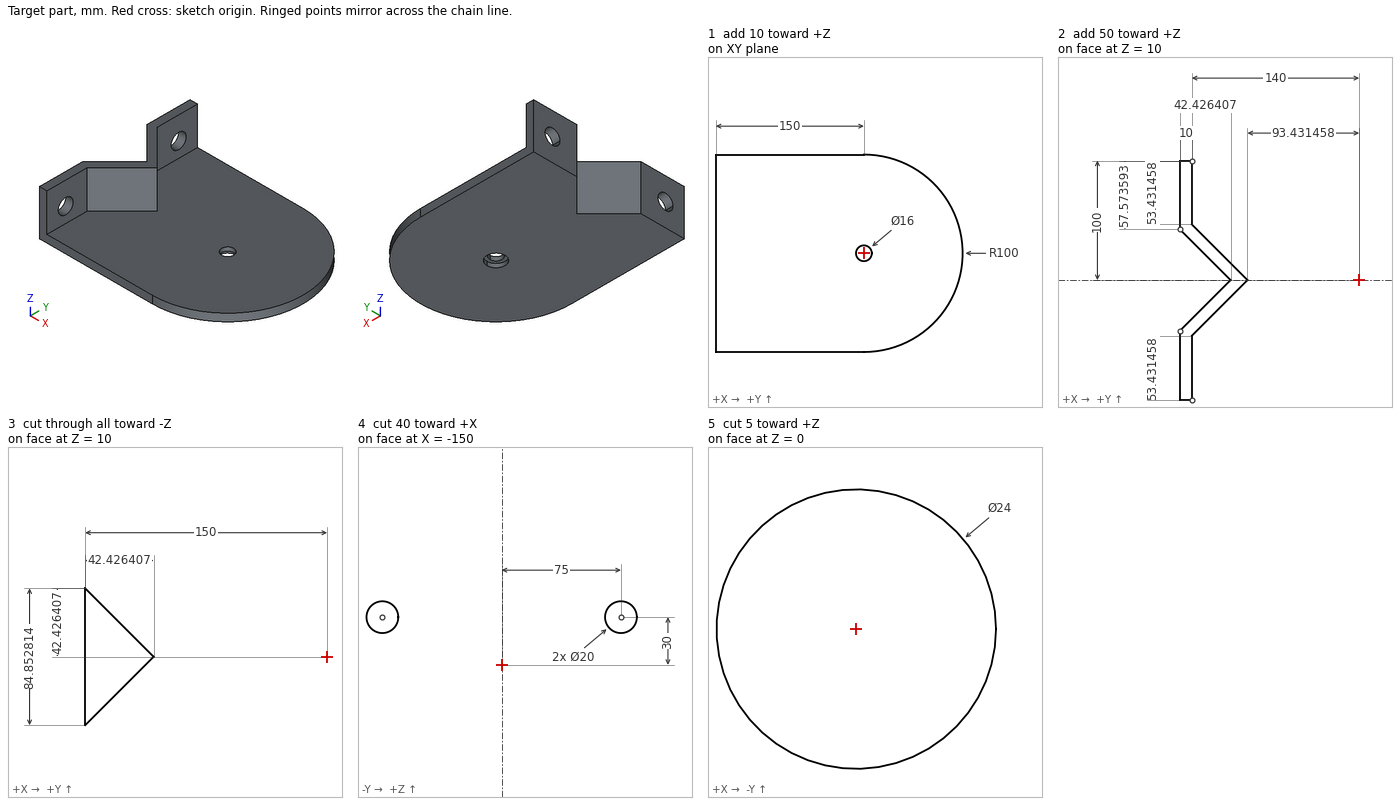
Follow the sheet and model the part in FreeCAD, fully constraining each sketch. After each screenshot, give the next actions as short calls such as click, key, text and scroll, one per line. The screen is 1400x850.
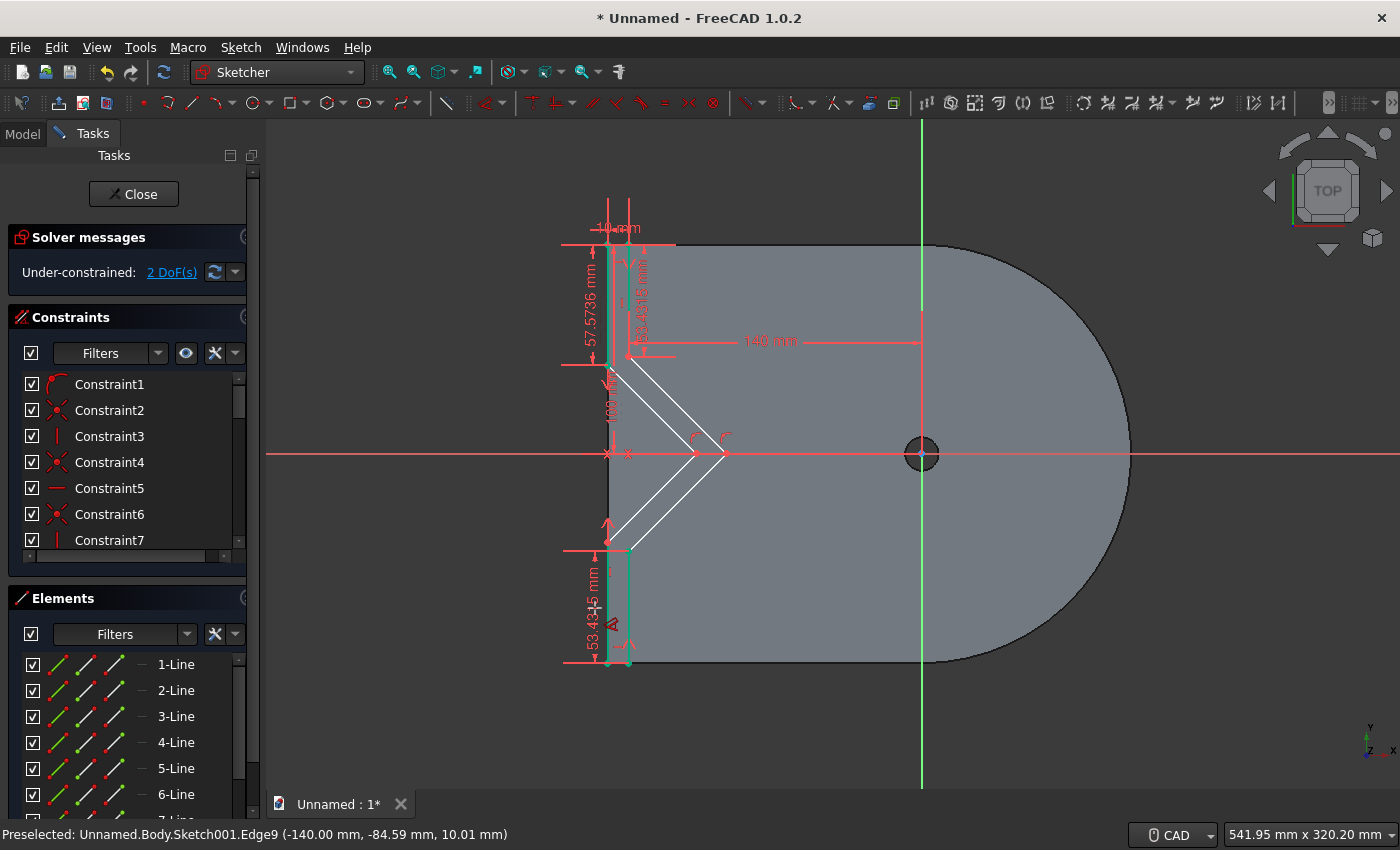
click(726, 454)
click(824, 488)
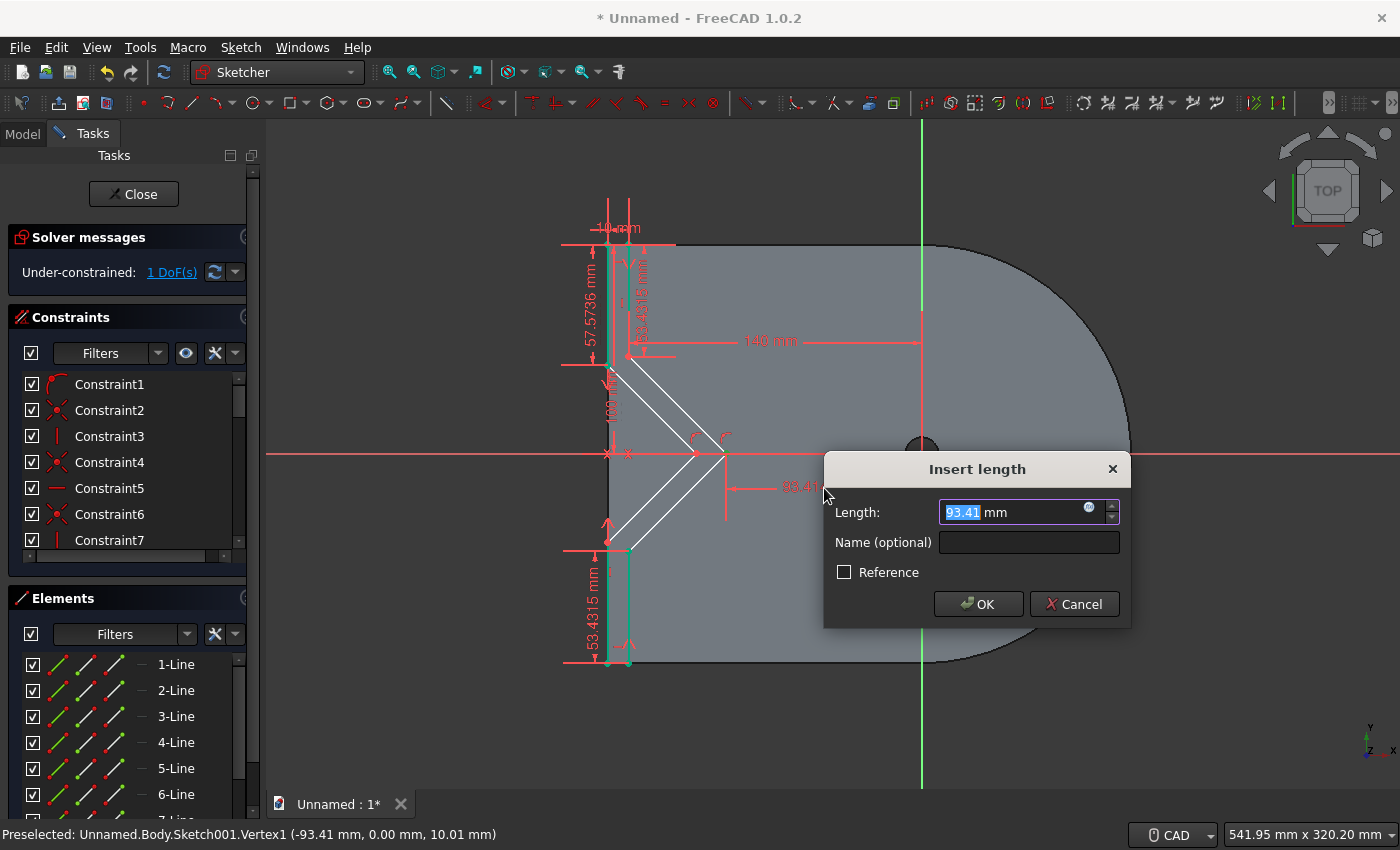
text(93.431458)
key(Return)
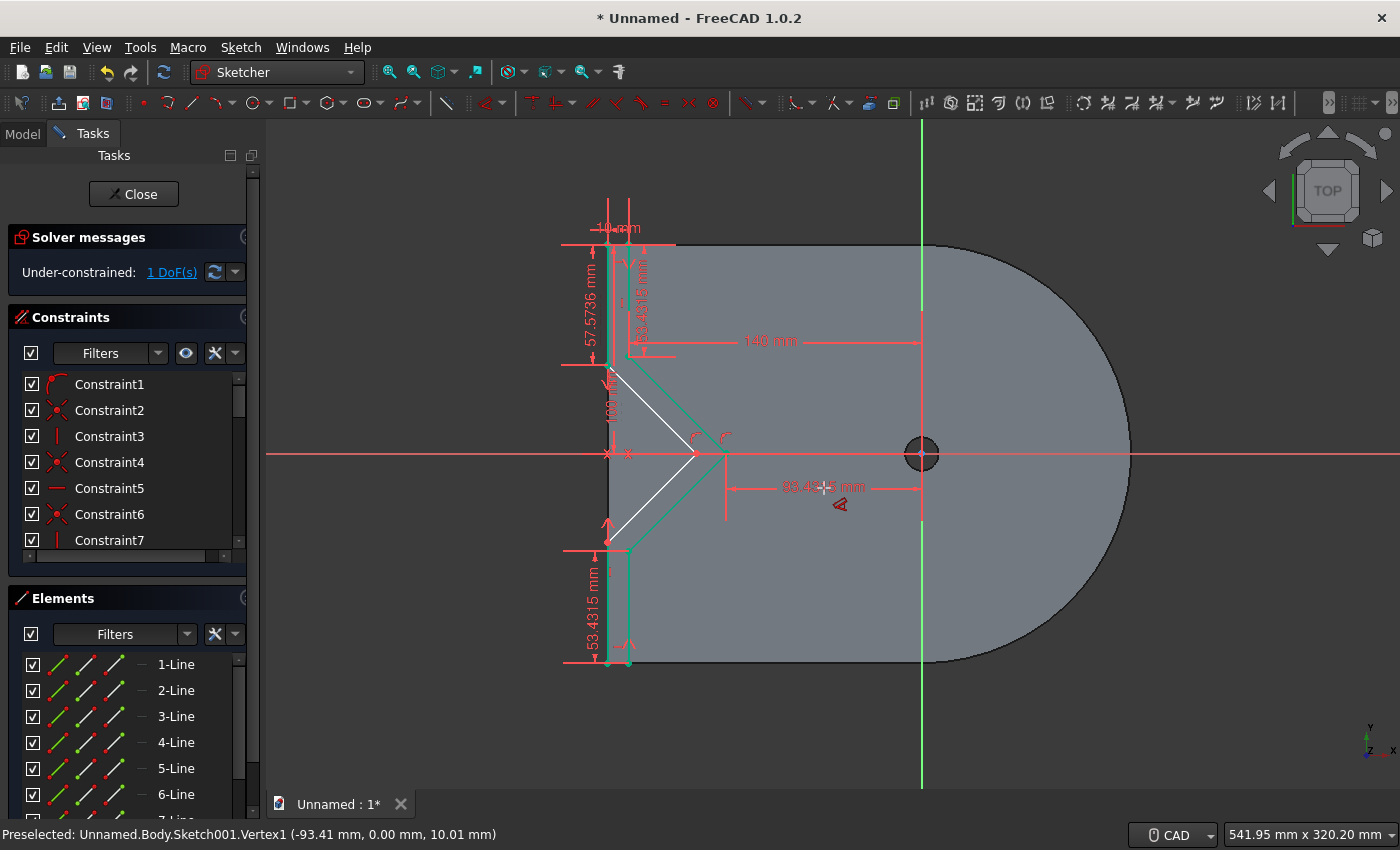
click(634, 392)
click(652, 331)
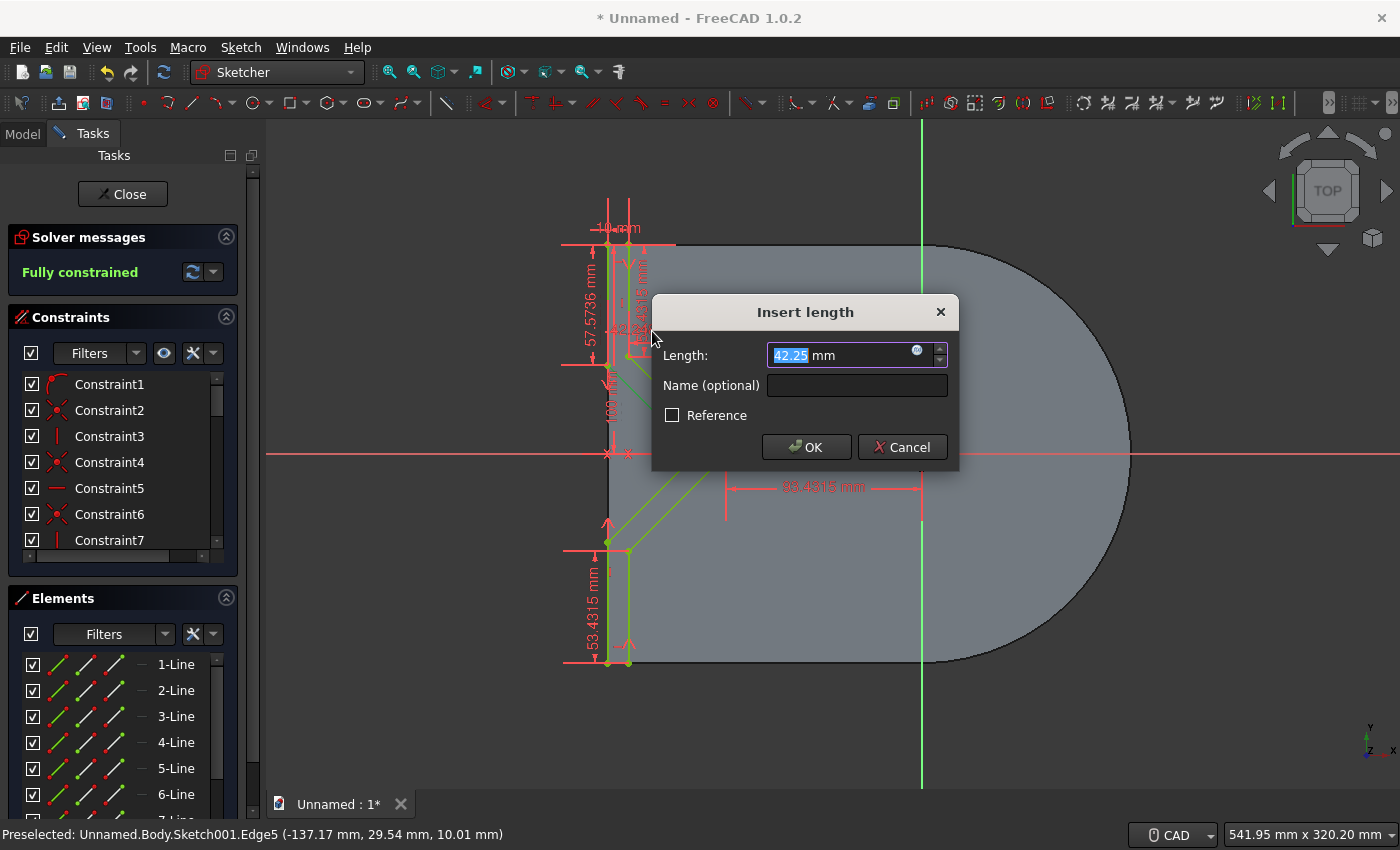
text(42.426407)
key(Return)
key(Escape)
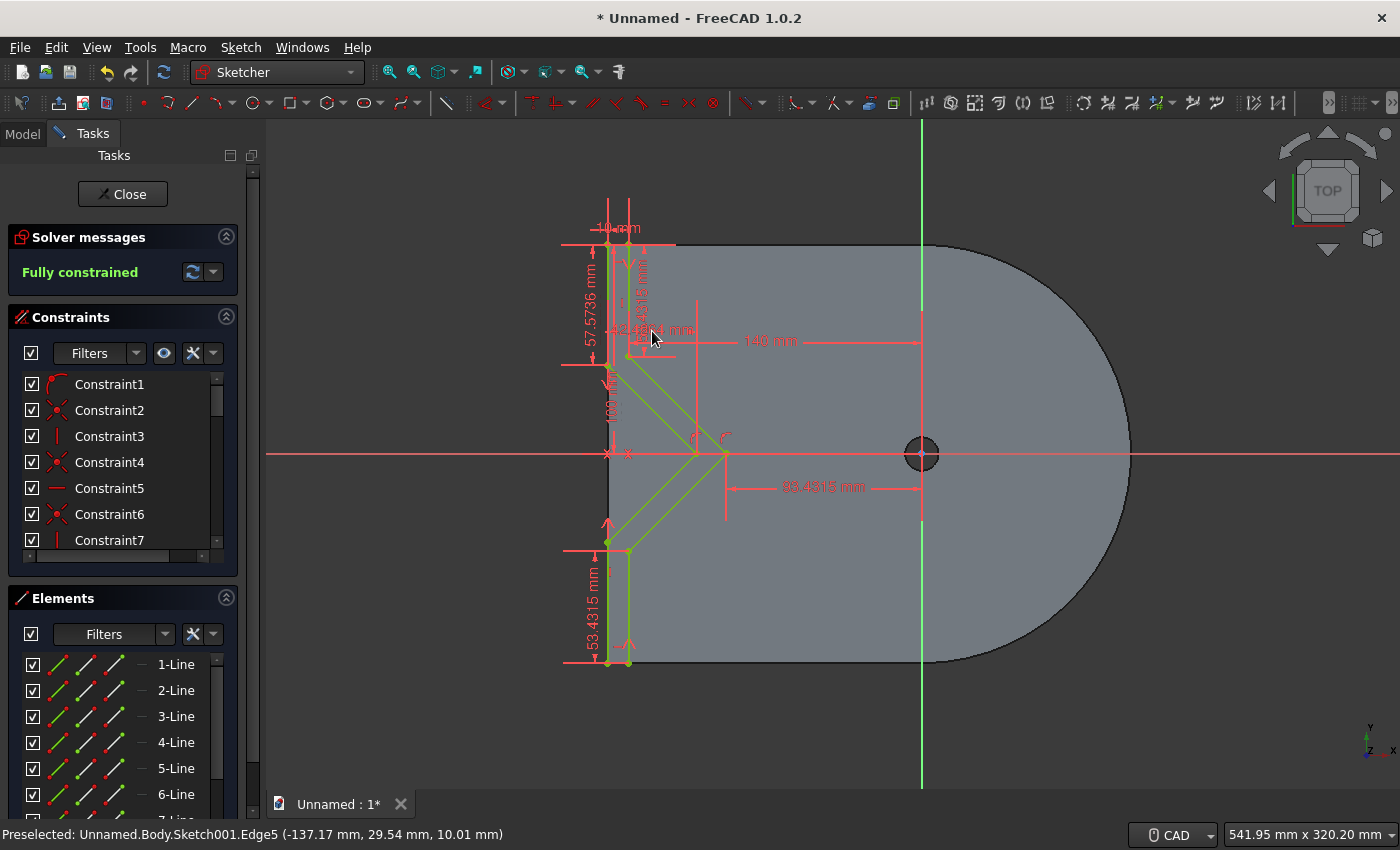
click(123, 194)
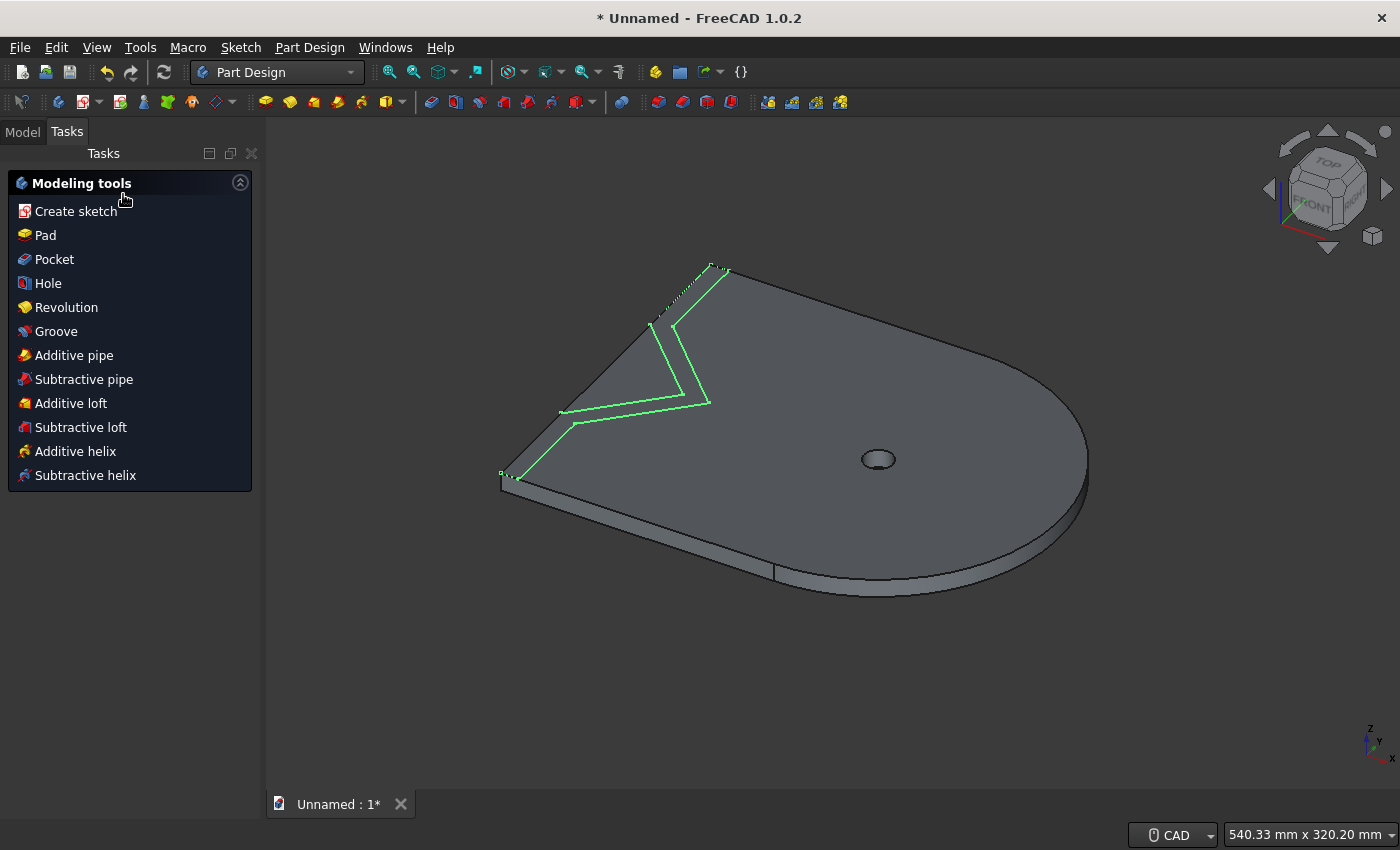
click(266, 102)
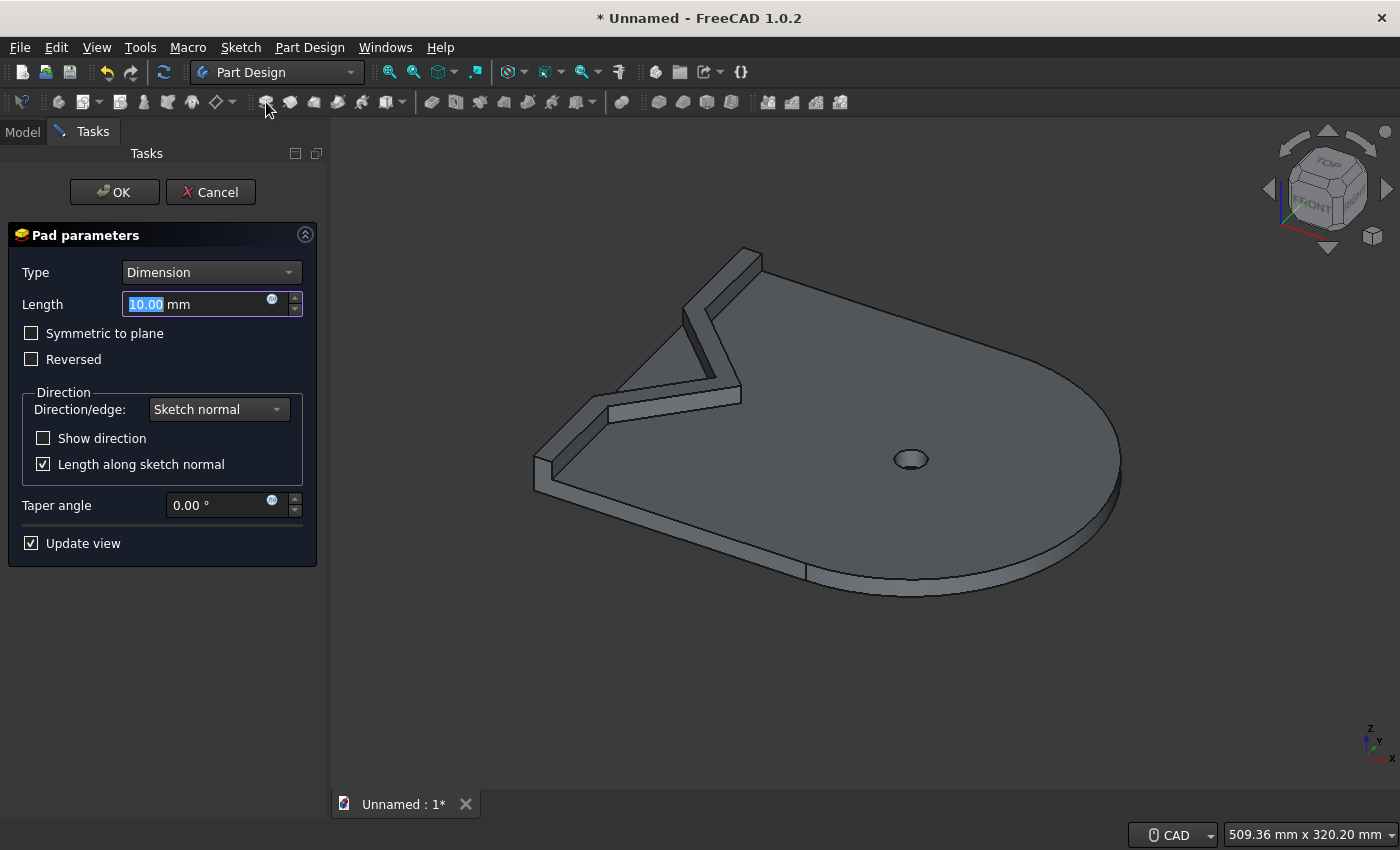
text(50)
key(Tab)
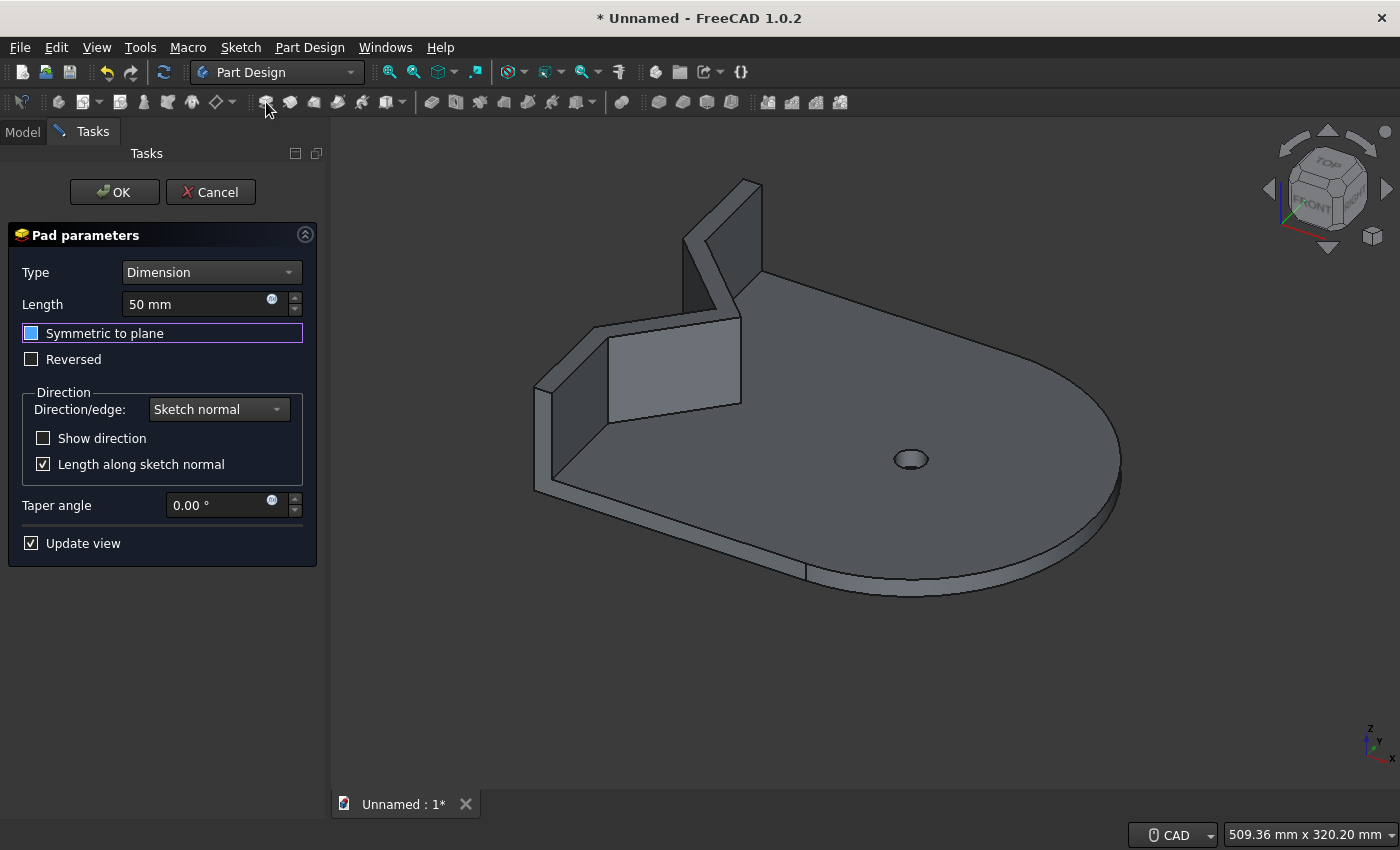
click(115, 192)